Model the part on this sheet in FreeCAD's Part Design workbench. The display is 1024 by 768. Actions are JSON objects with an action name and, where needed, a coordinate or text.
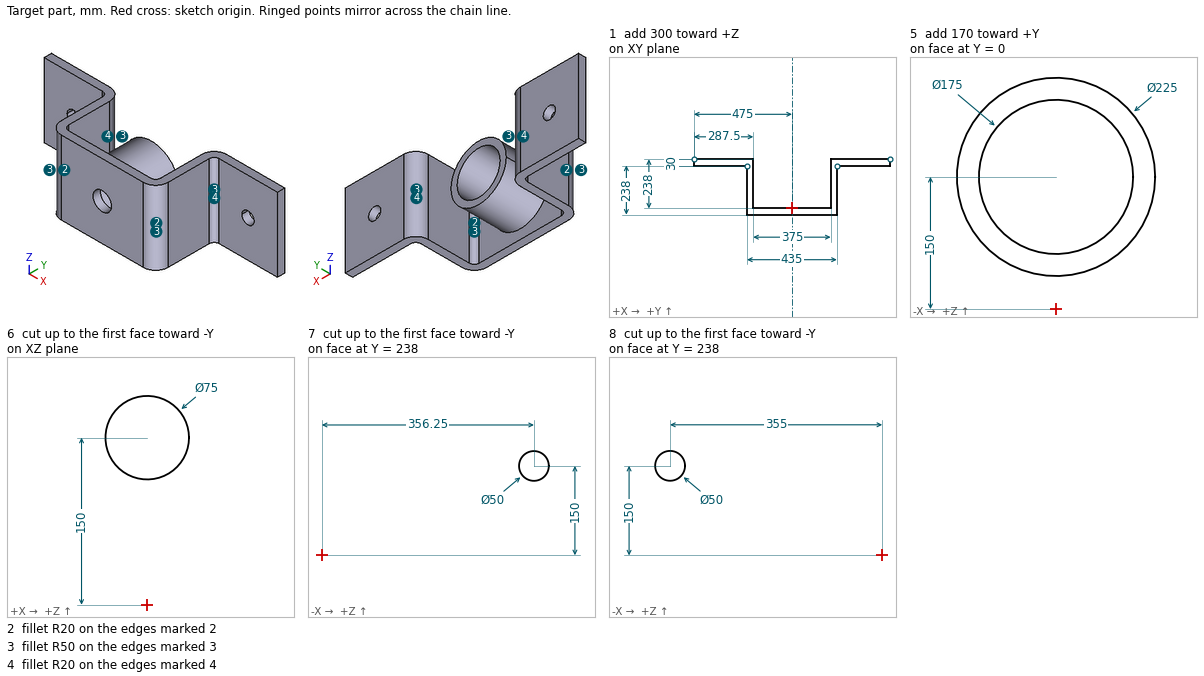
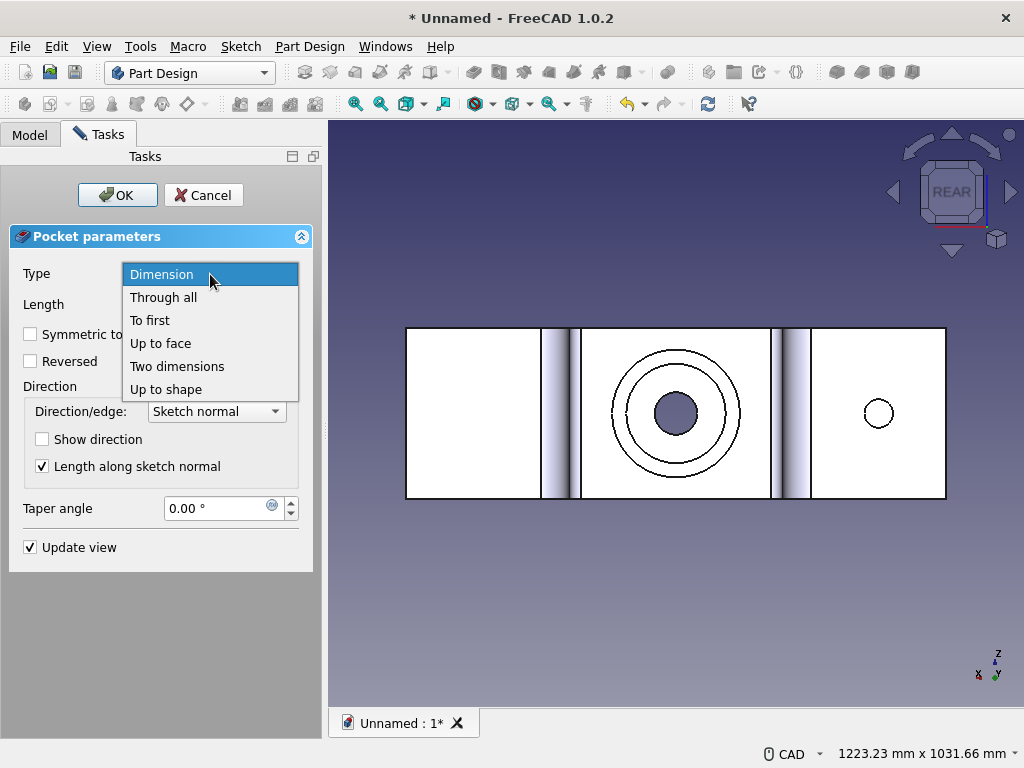
{"action": "left_click", "coordinate": [208, 320]}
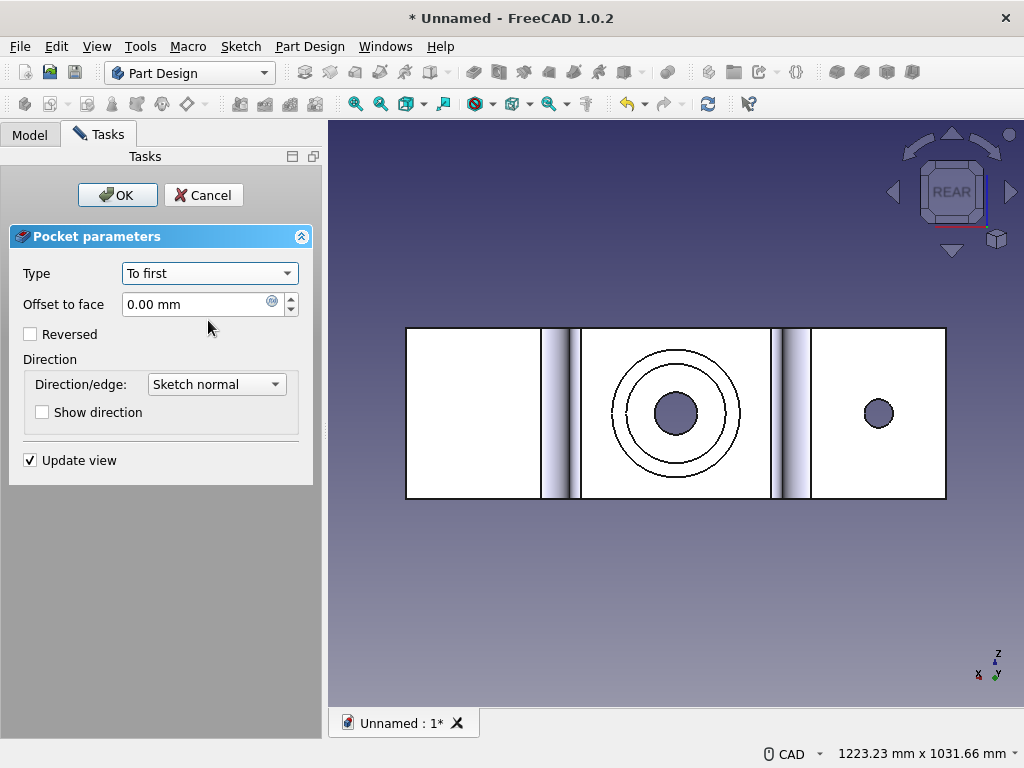
{"action": "left_click", "coordinate": [118, 195]}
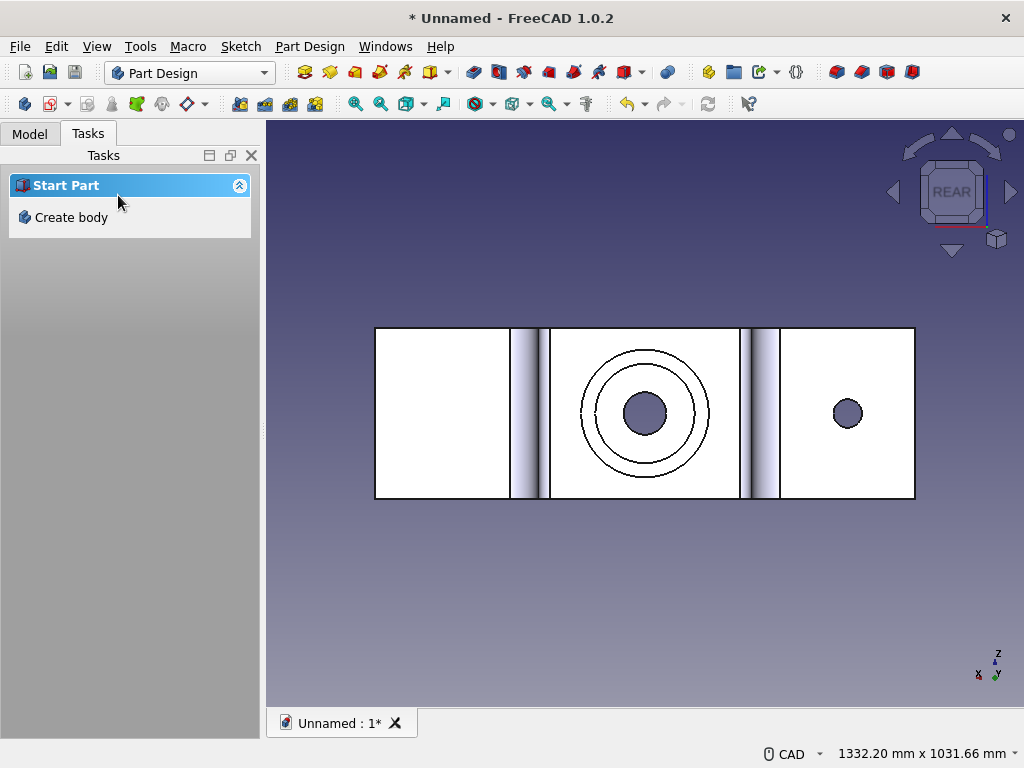
{"action": "left_click", "coordinate": [442, 412]}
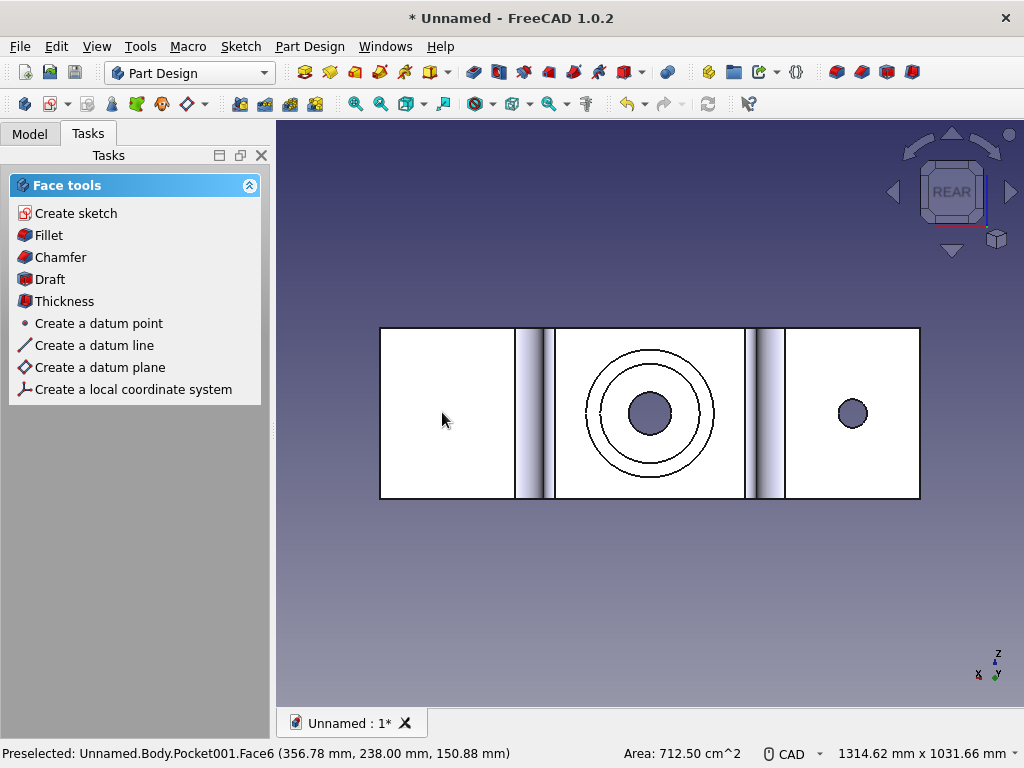
{"action": "left_click", "coordinate": [50, 104]}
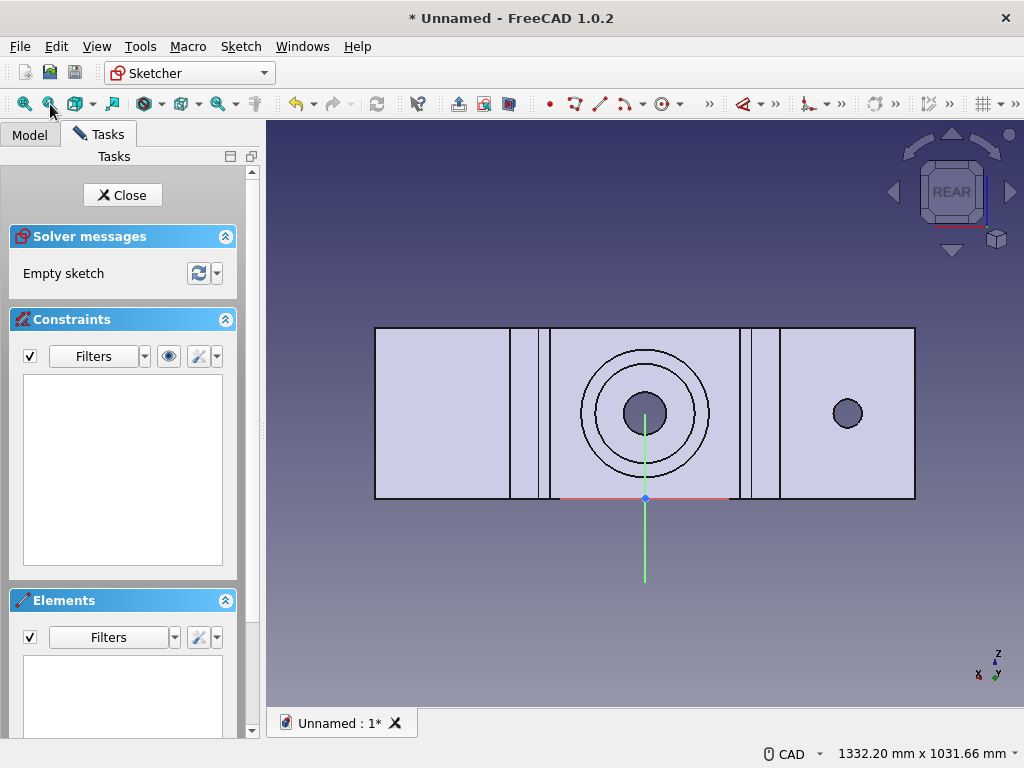
{"action": "scroll", "coordinate": [432, 414], "scroll_direction": "up", "scroll_amount": 13}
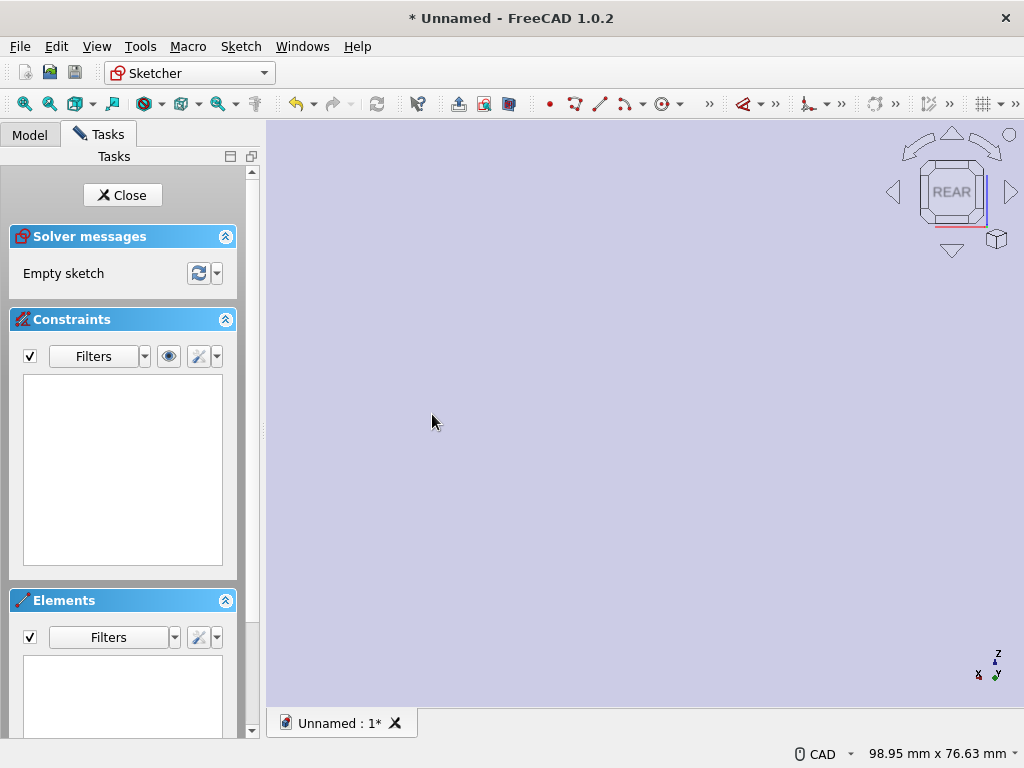
{"action": "left_click", "coordinate": [662, 104]}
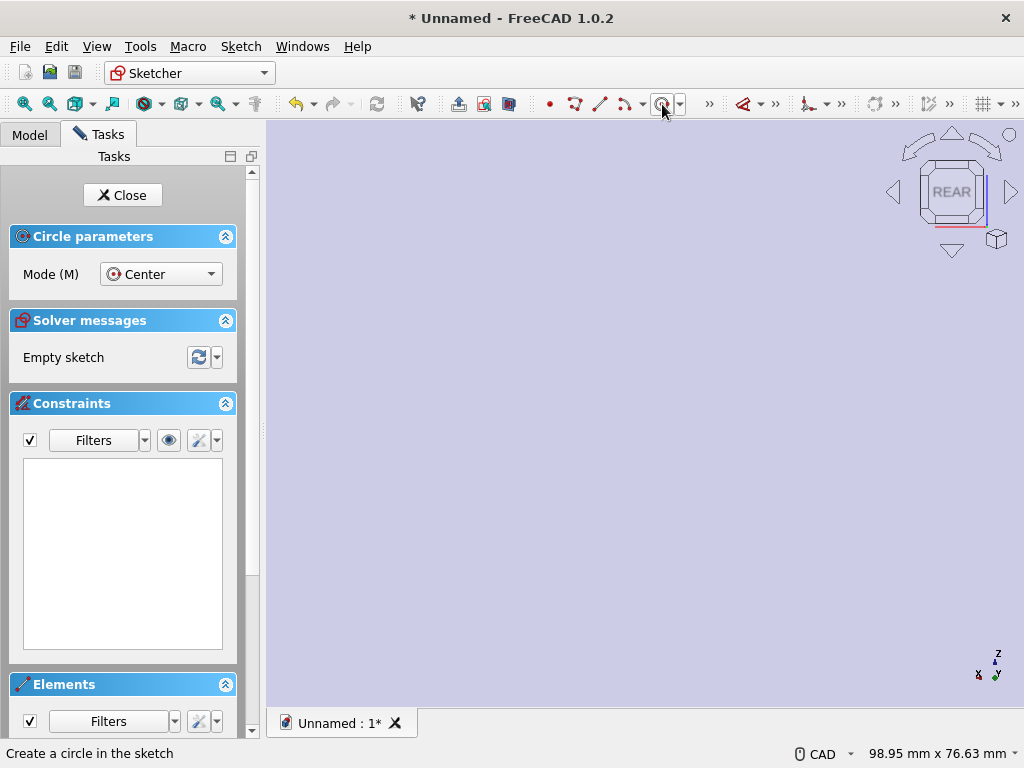
{"action": "left_click", "coordinate": [578, 401]}
{"action": "left_click", "coordinate": [713, 266]}
{"action": "key", "text": "Escape"}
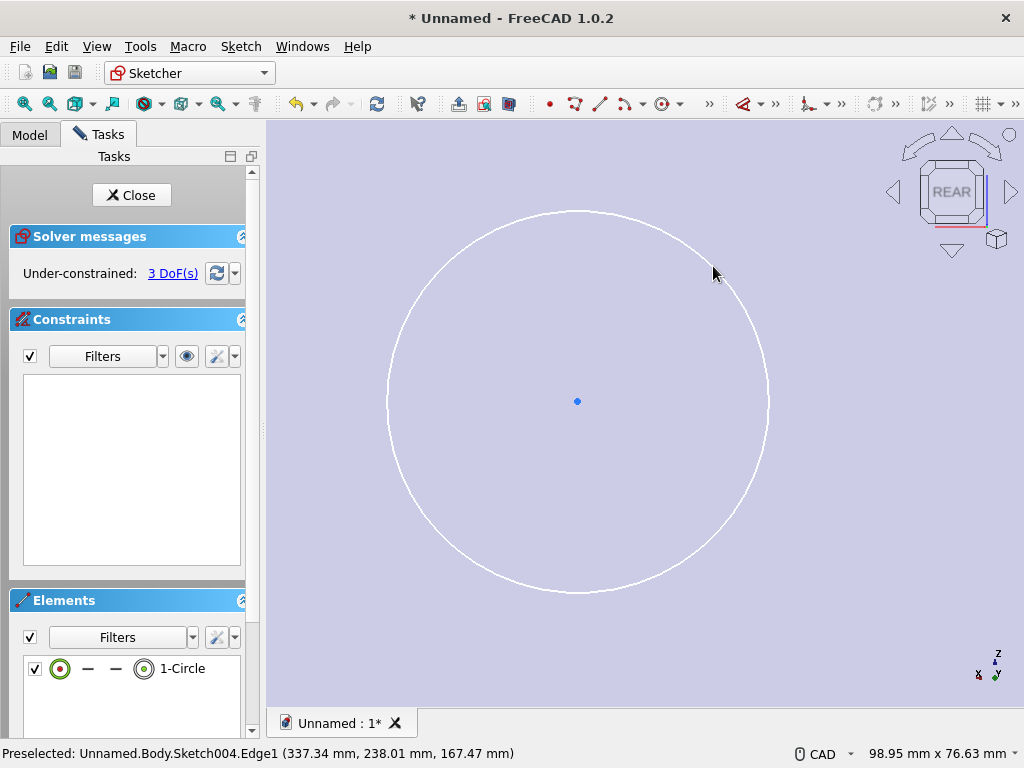
{"action": "left_click", "coordinate": [742, 104]}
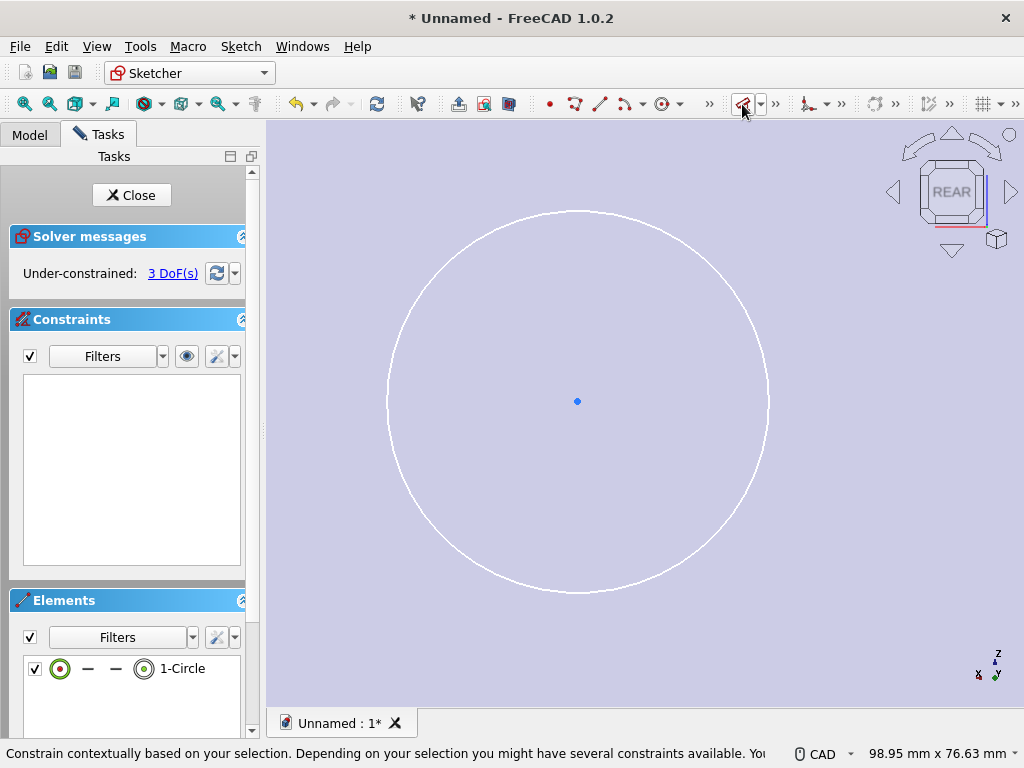
{"action": "left_click", "coordinate": [713, 267]}
{"action": "left_click", "coordinate": [736, 244]}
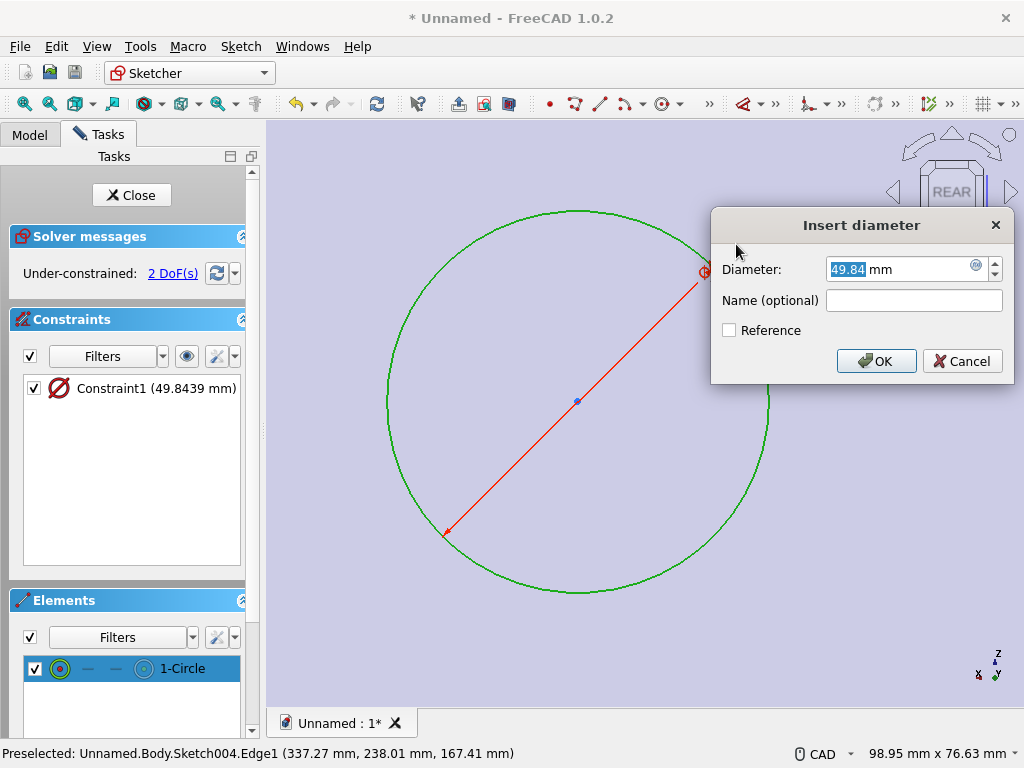
{"action": "type", "text": "50"}
{"action": "key", "text": "Return"}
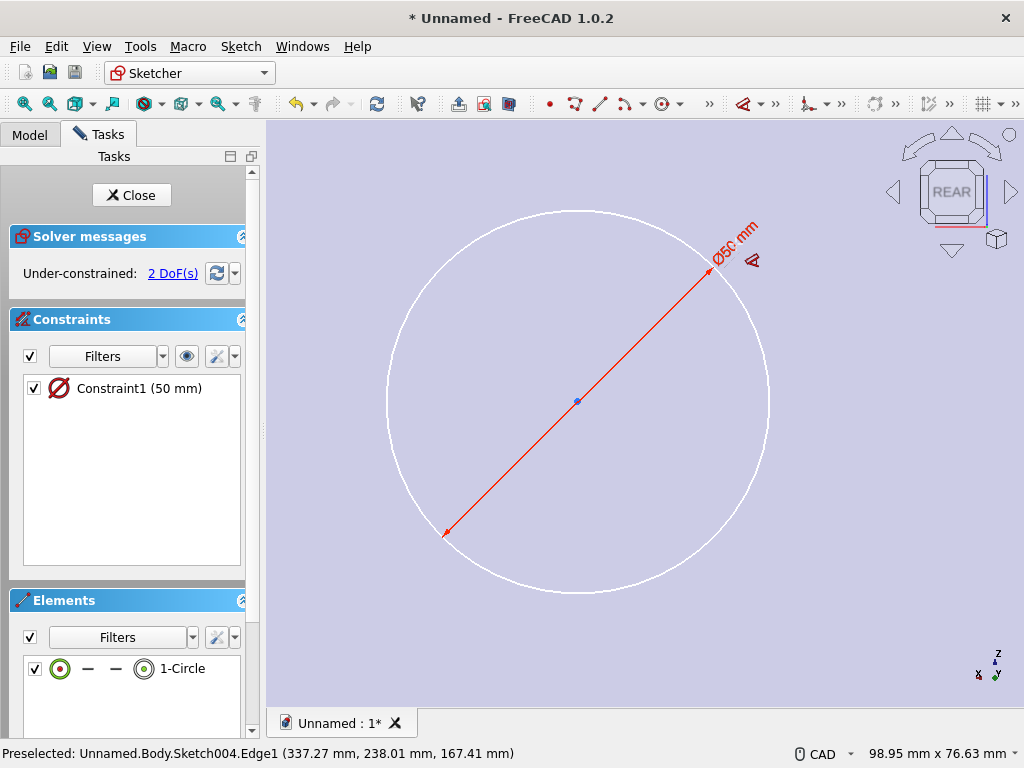
{"action": "left_click", "coordinate": [578, 402]}
{"action": "left_click", "coordinate": [719, 368]}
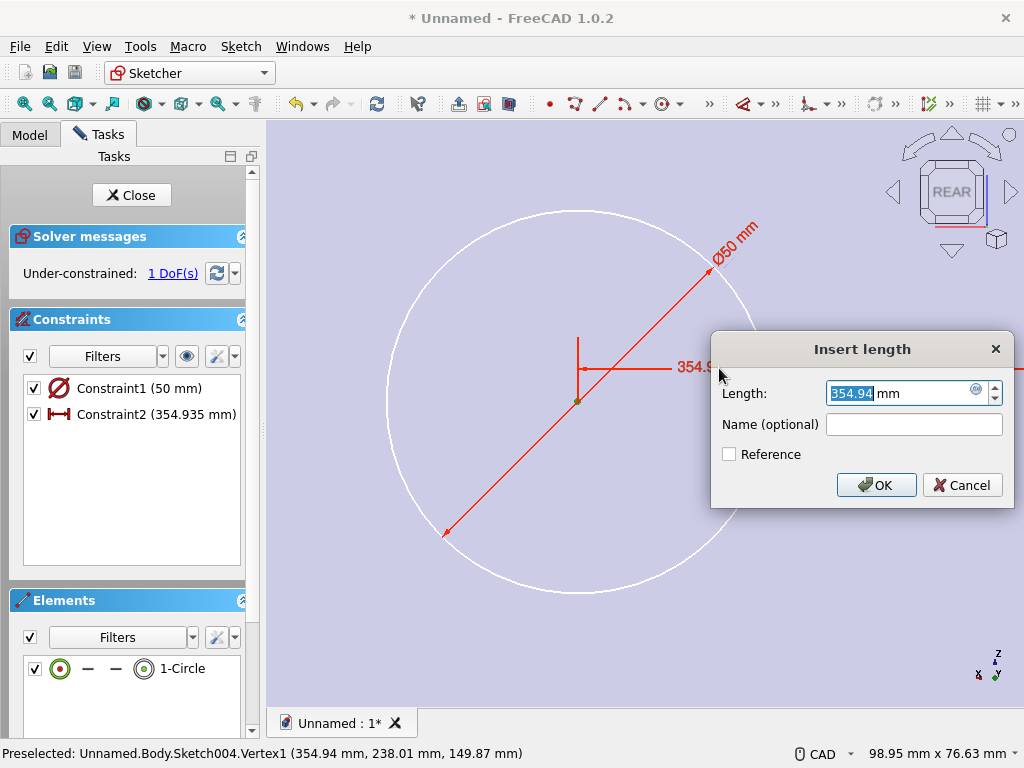
{"action": "type", "text": "355"}
{"action": "key", "text": "Return"}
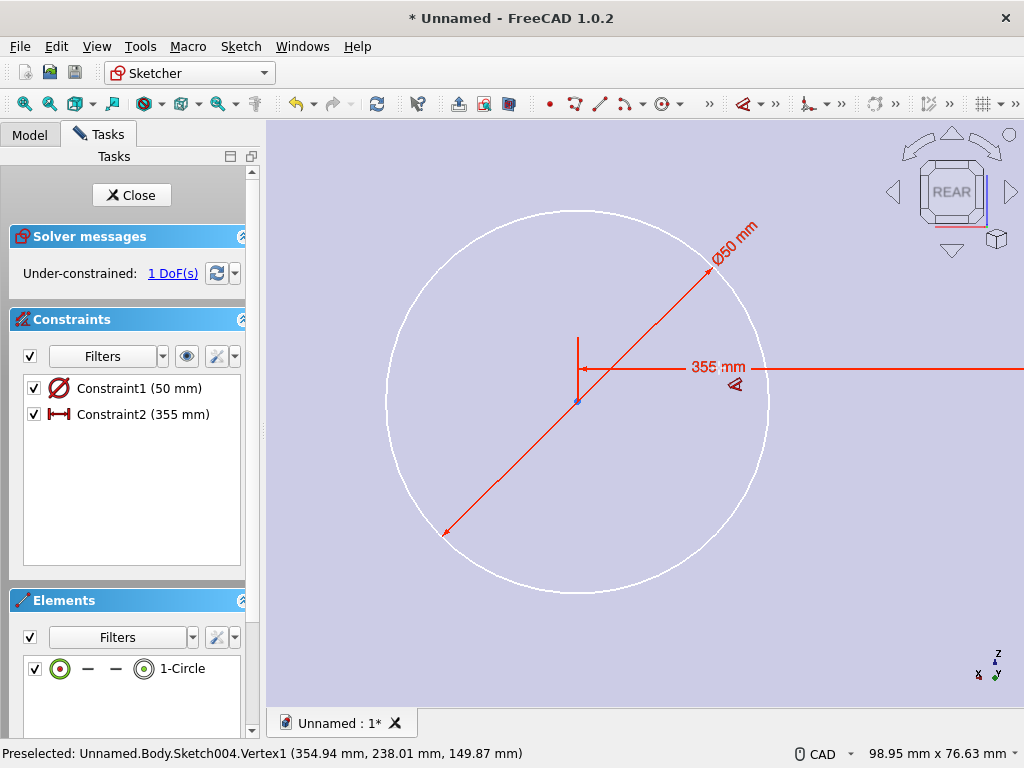
{"action": "left_click", "coordinate": [578, 402]}
{"action": "left_click", "coordinate": [544, 540]}